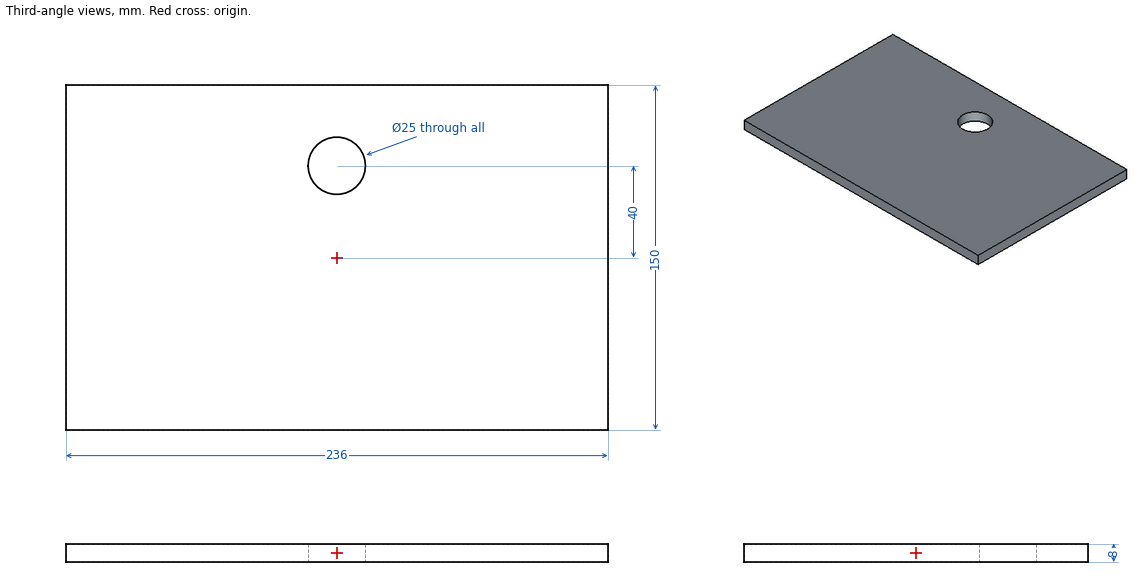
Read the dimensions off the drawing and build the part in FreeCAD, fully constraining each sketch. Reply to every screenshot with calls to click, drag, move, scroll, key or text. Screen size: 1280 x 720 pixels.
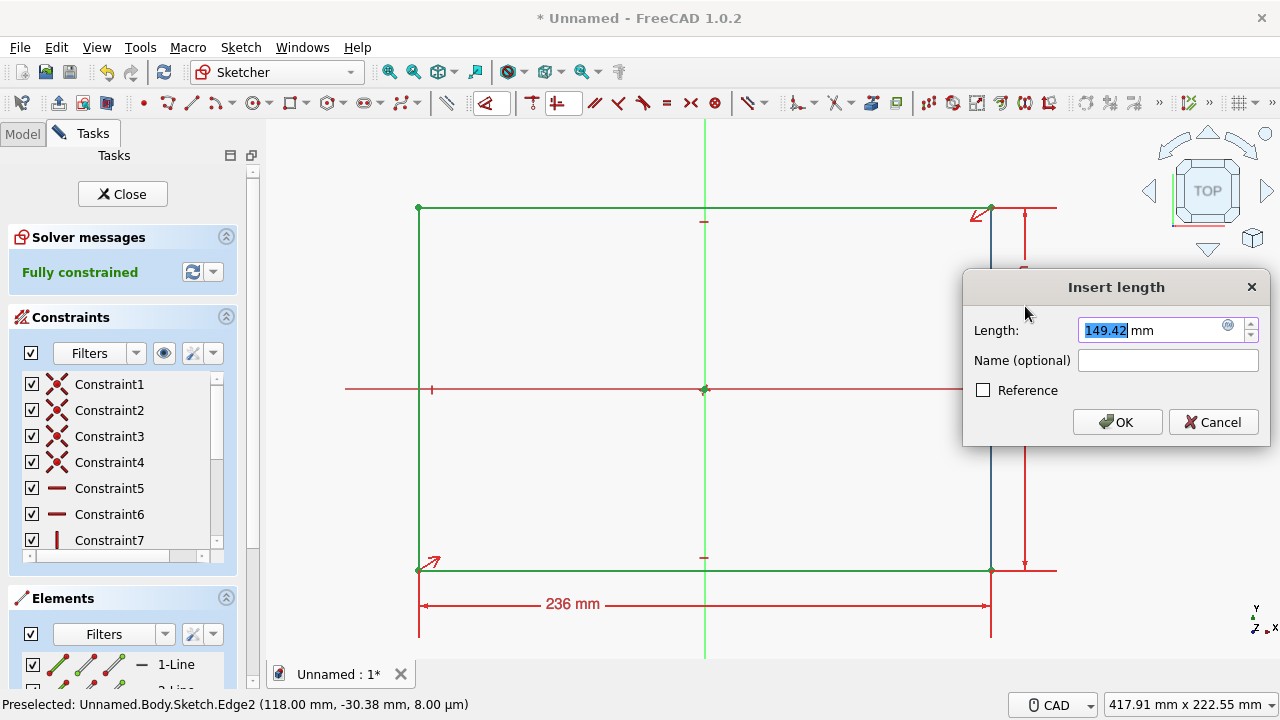
text(150)
key(Return)
key(Escape)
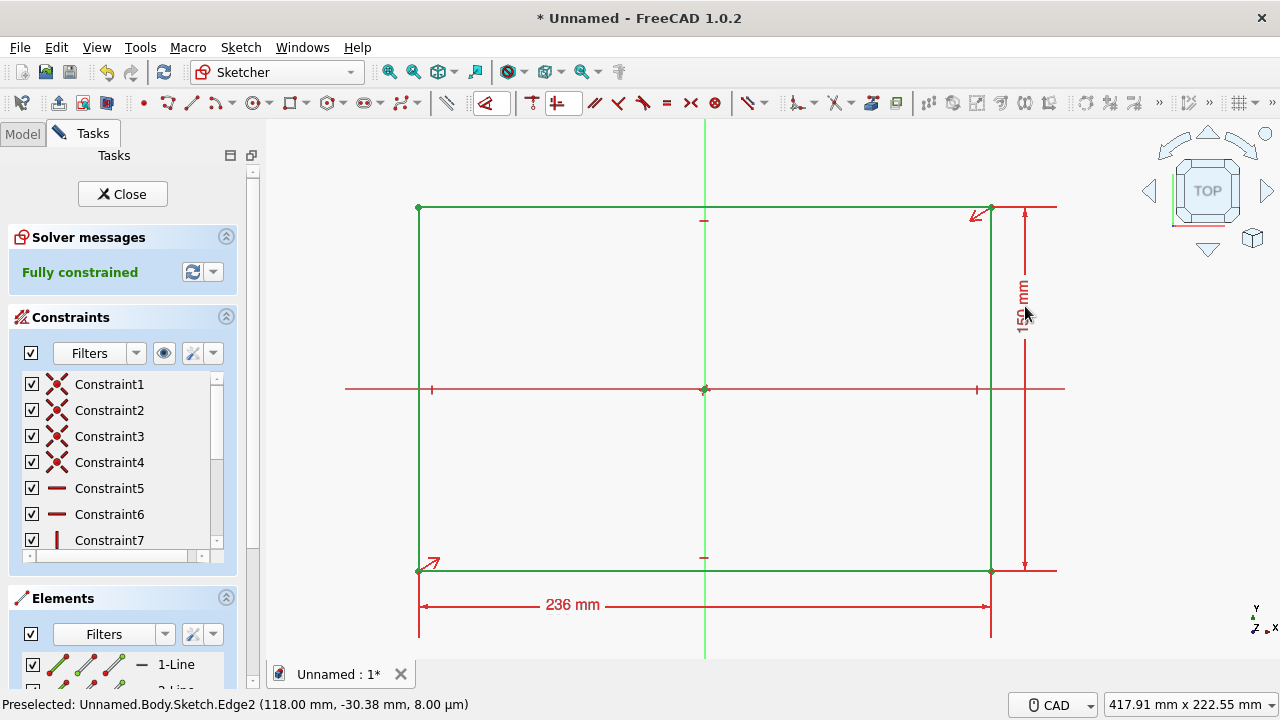
click(123, 194)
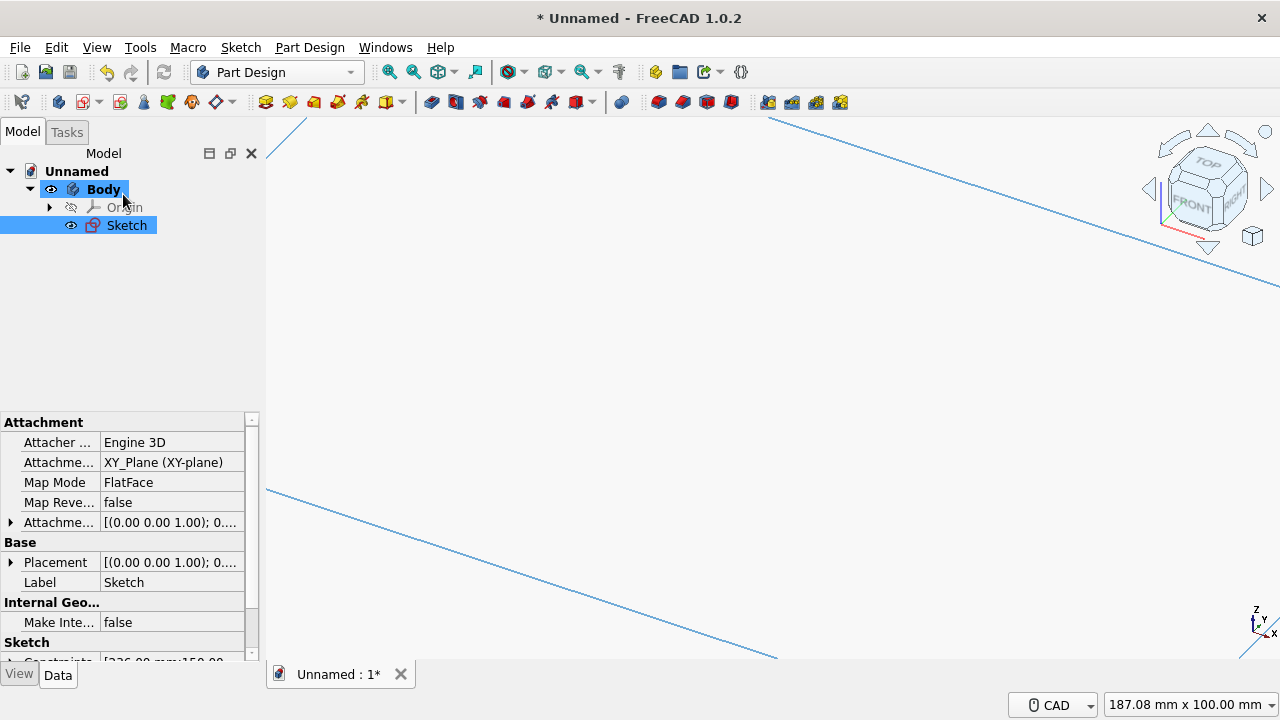
click(266, 102)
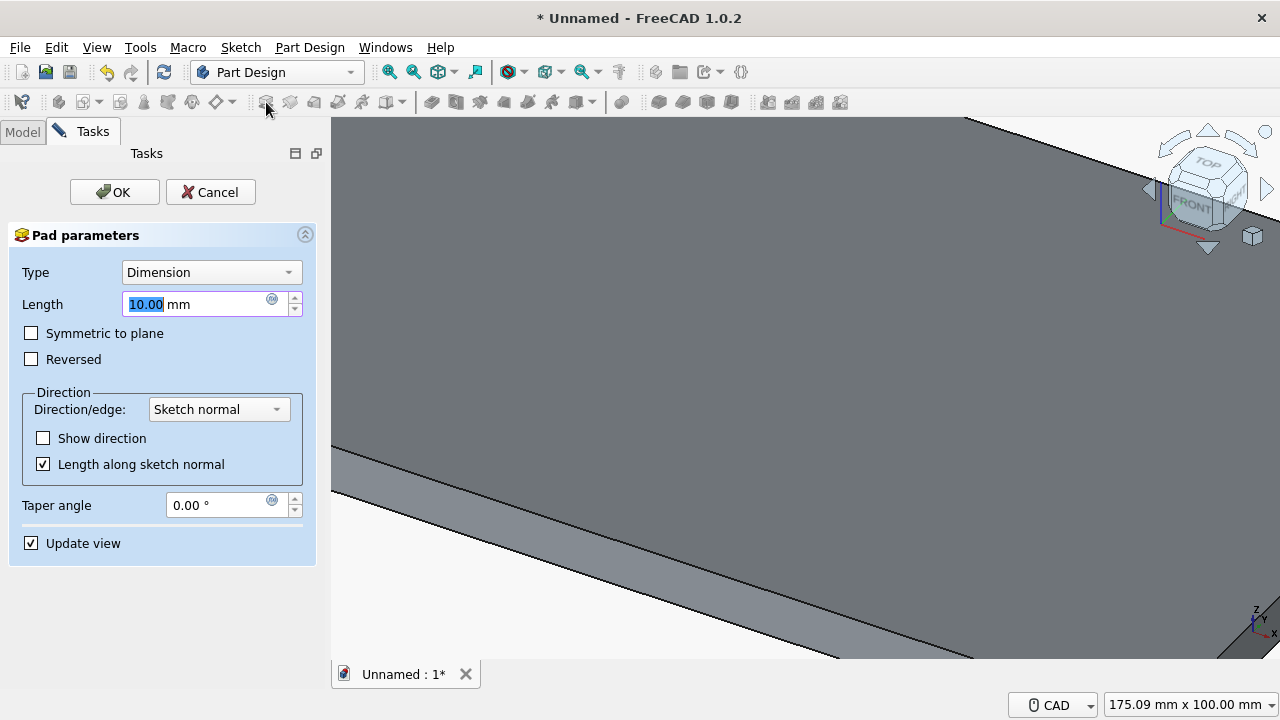
text(8)
key(Tab)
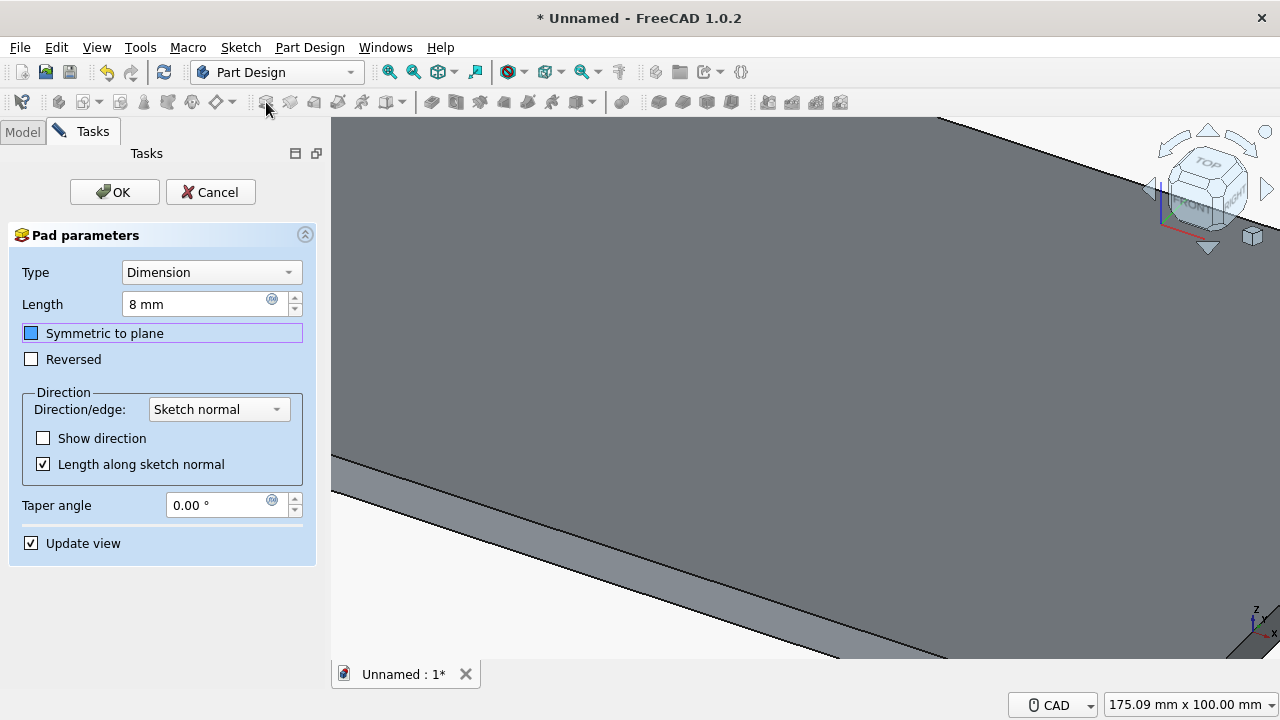
click(30, 333)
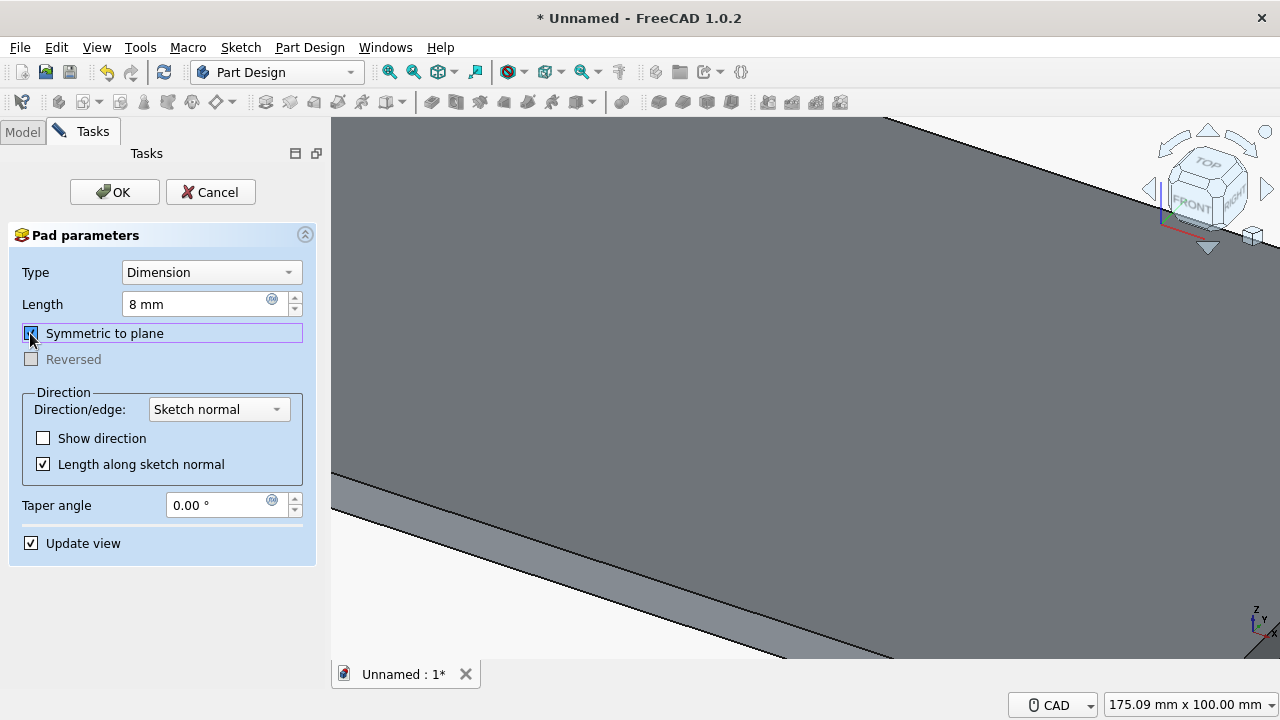
click(115, 192)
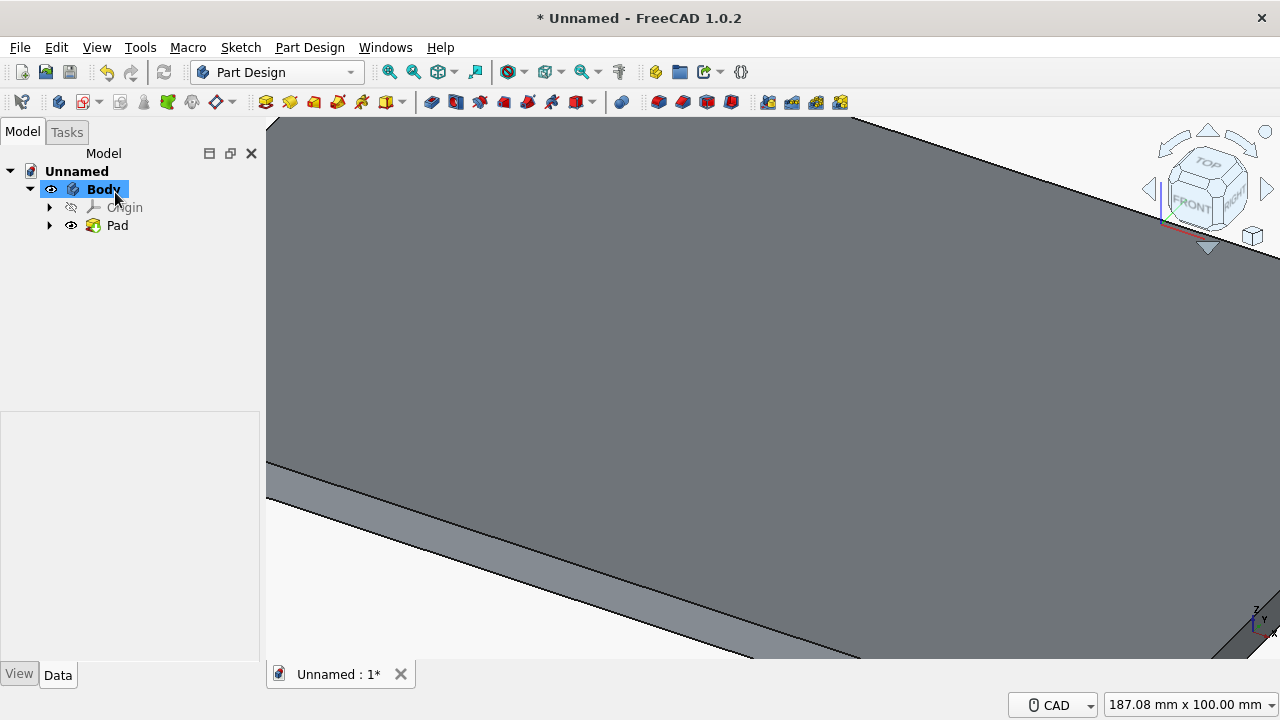
click(390, 72)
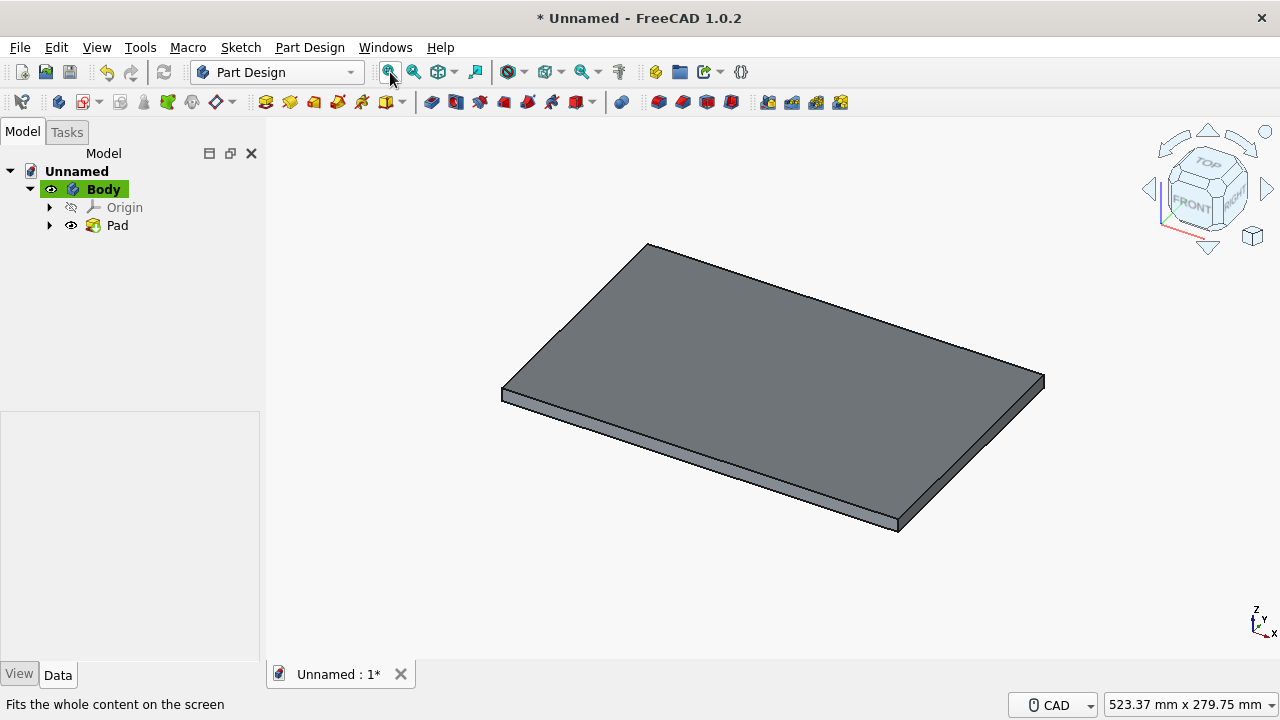
click(830, 399)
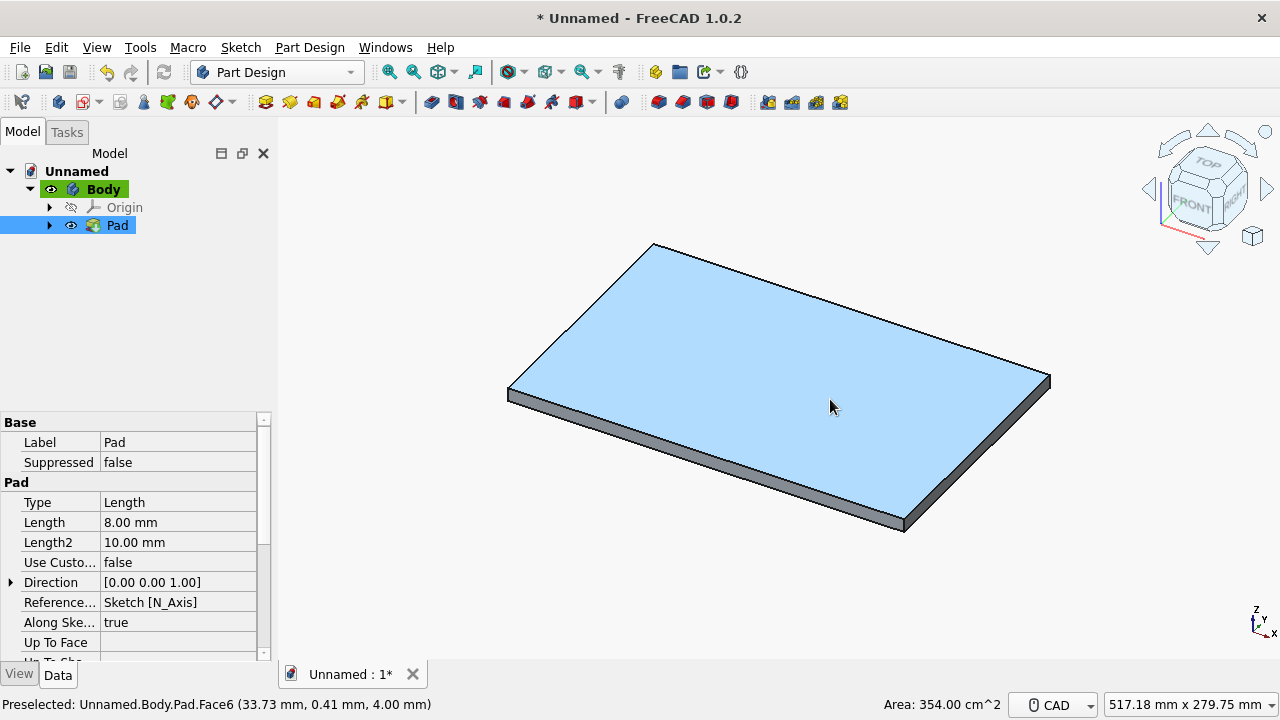
click(84, 102)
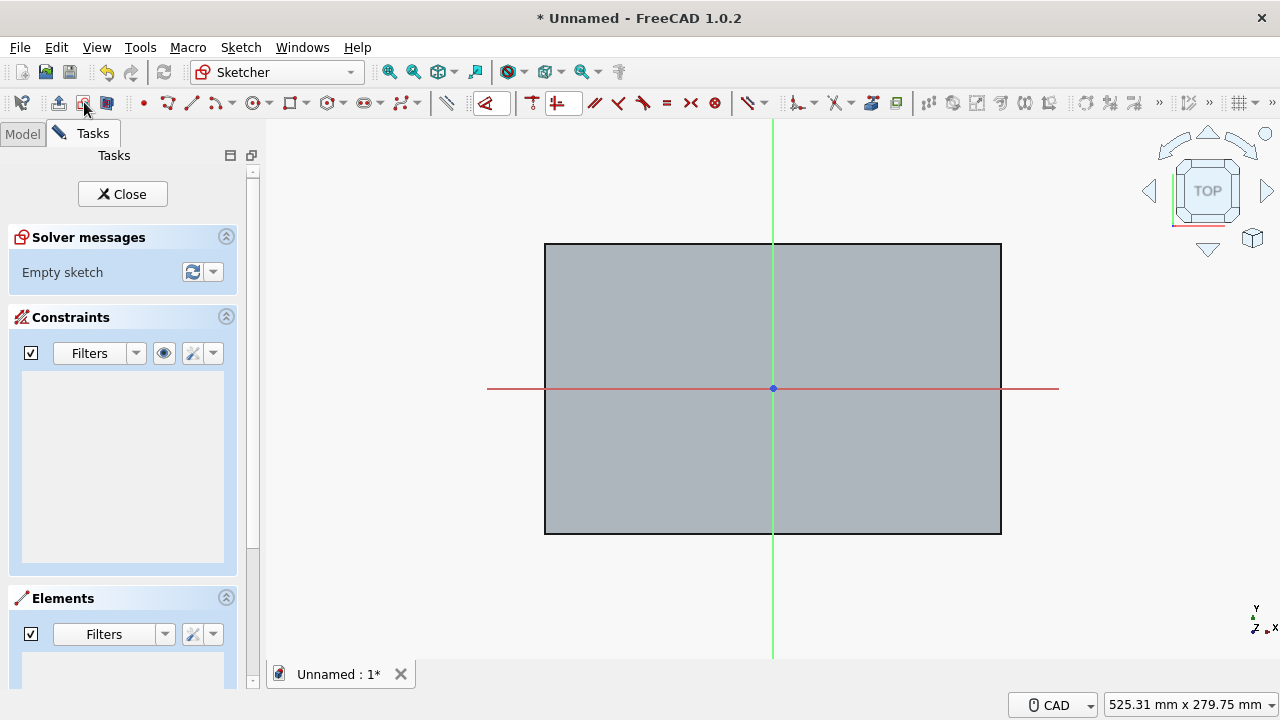
scroll(803, 316, up, 6)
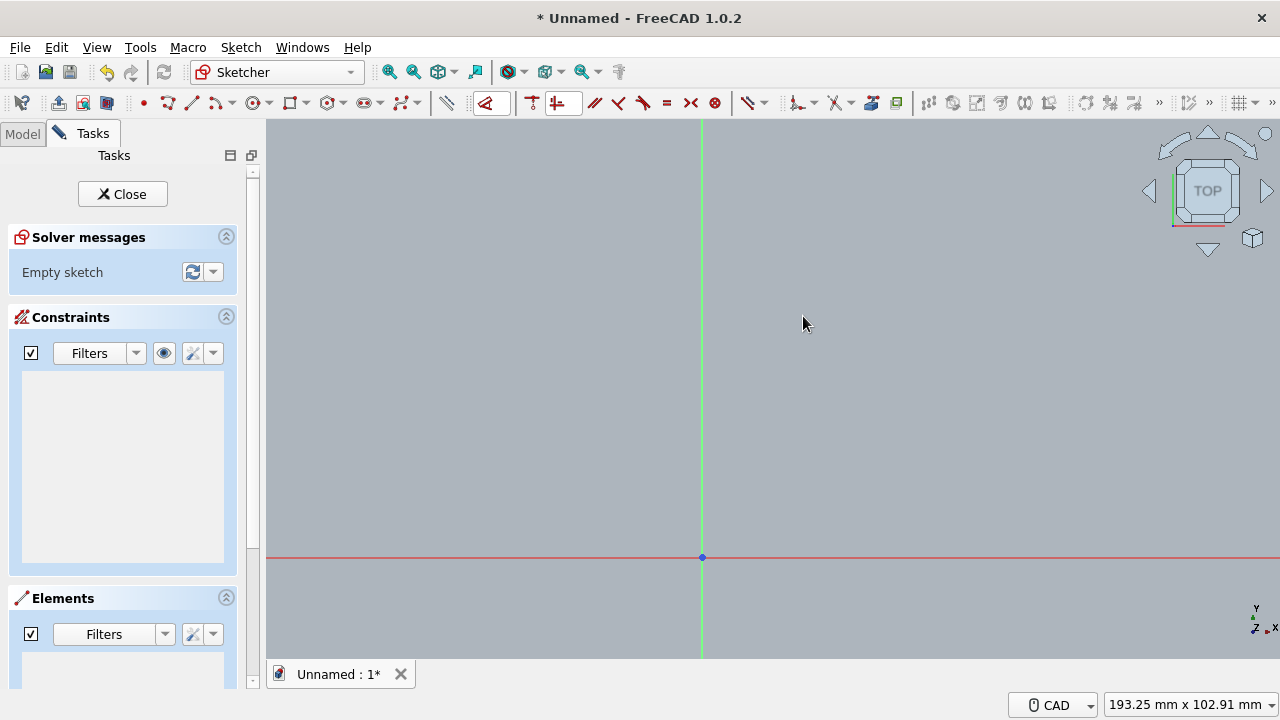
click(254, 104)